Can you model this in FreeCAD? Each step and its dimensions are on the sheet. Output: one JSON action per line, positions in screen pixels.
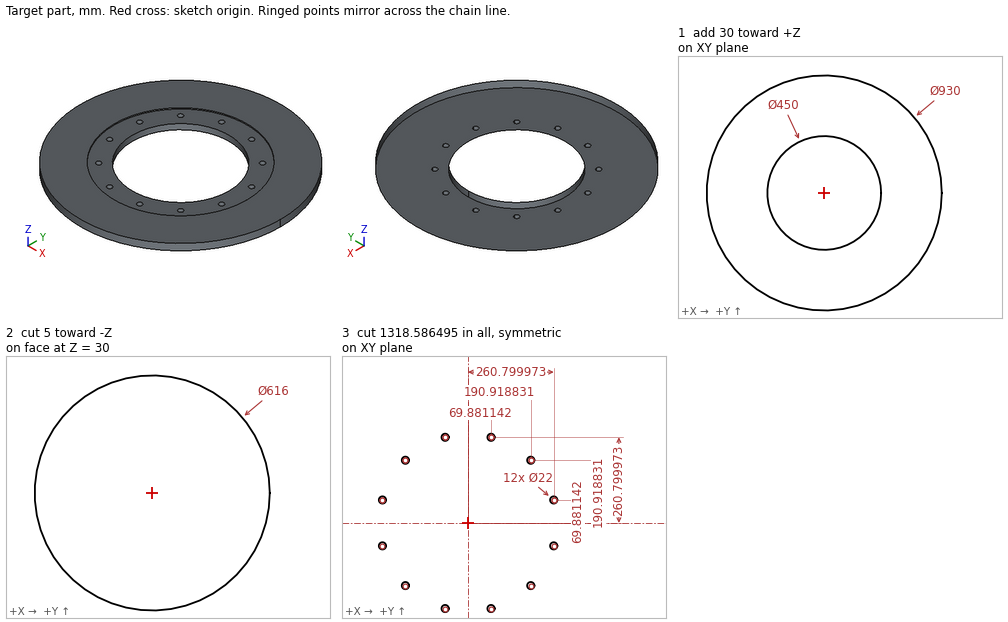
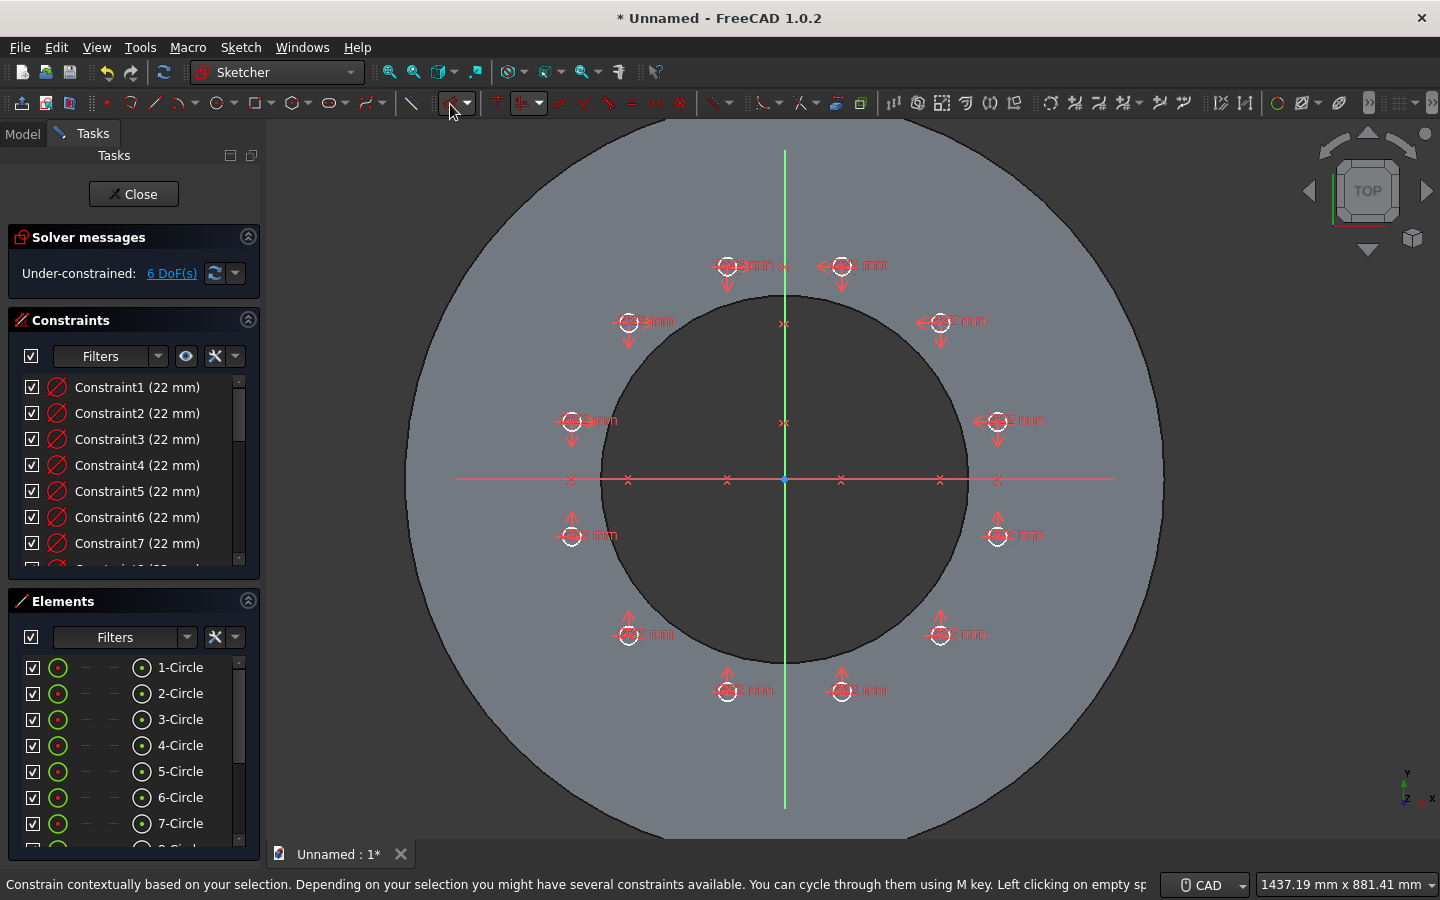
{"action": "left_click", "coordinate": [998, 422]}
{"action": "left_click", "coordinate": [1032, 451]}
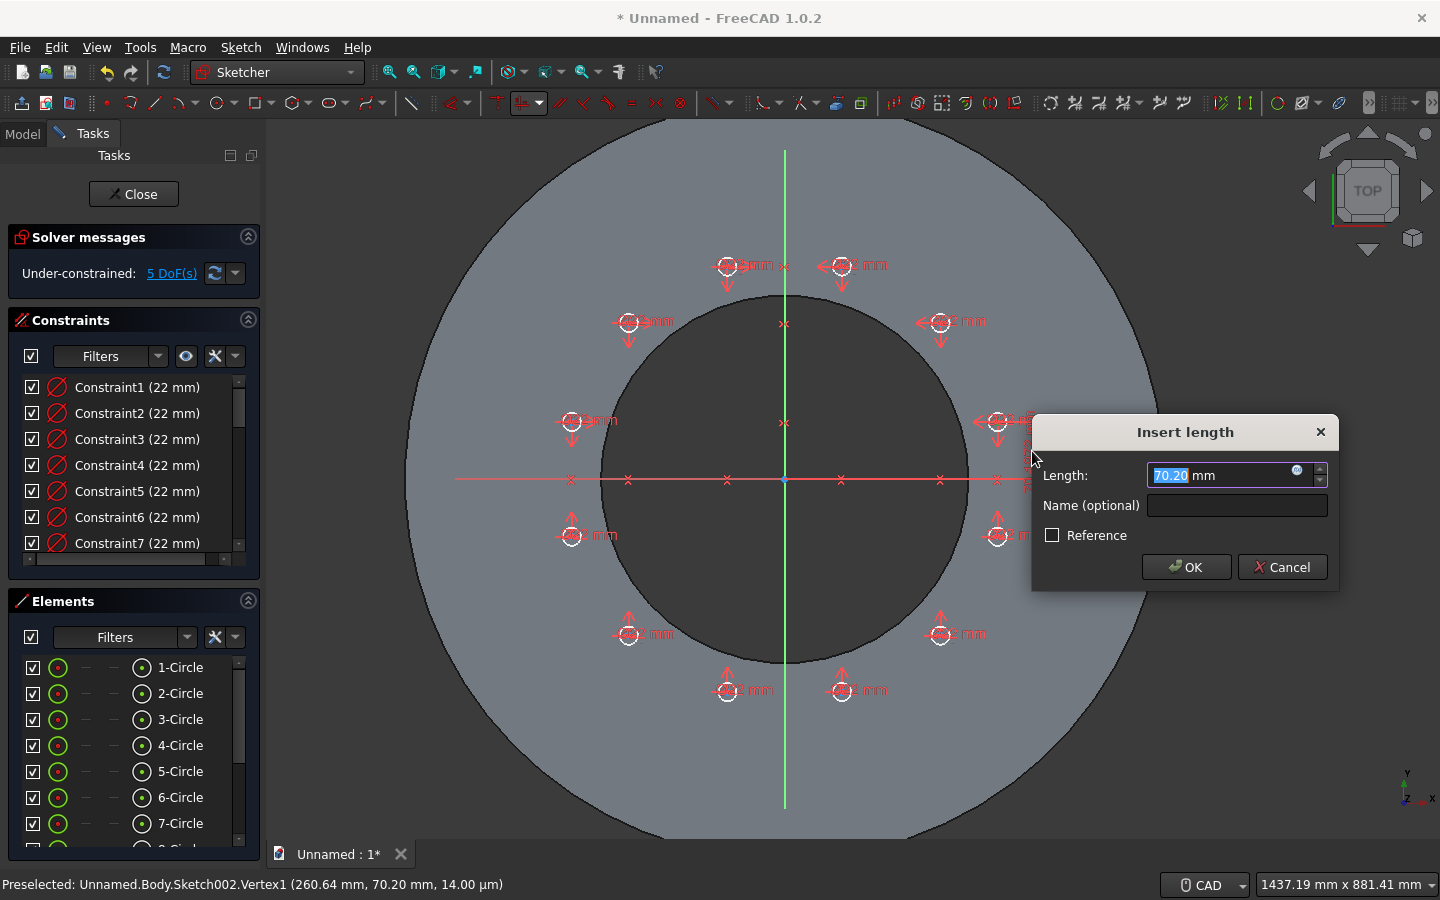
{"action": "type", "text": "69.881142"}
{"action": "key", "text": "Return"}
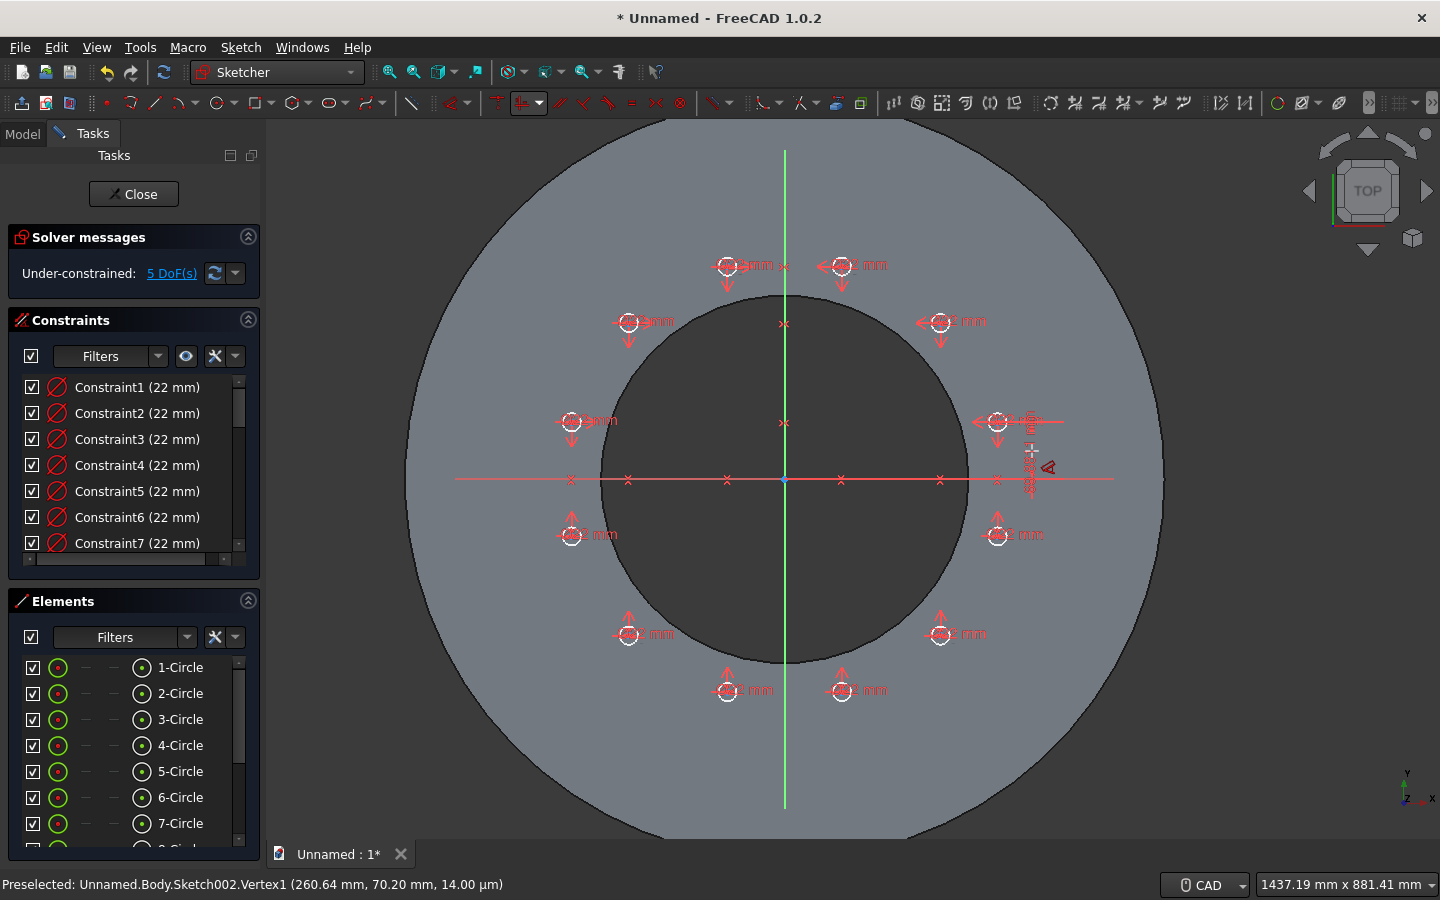
{"action": "left_click", "coordinate": [842, 267]}
{"action": "left_click", "coordinate": [813, 233]}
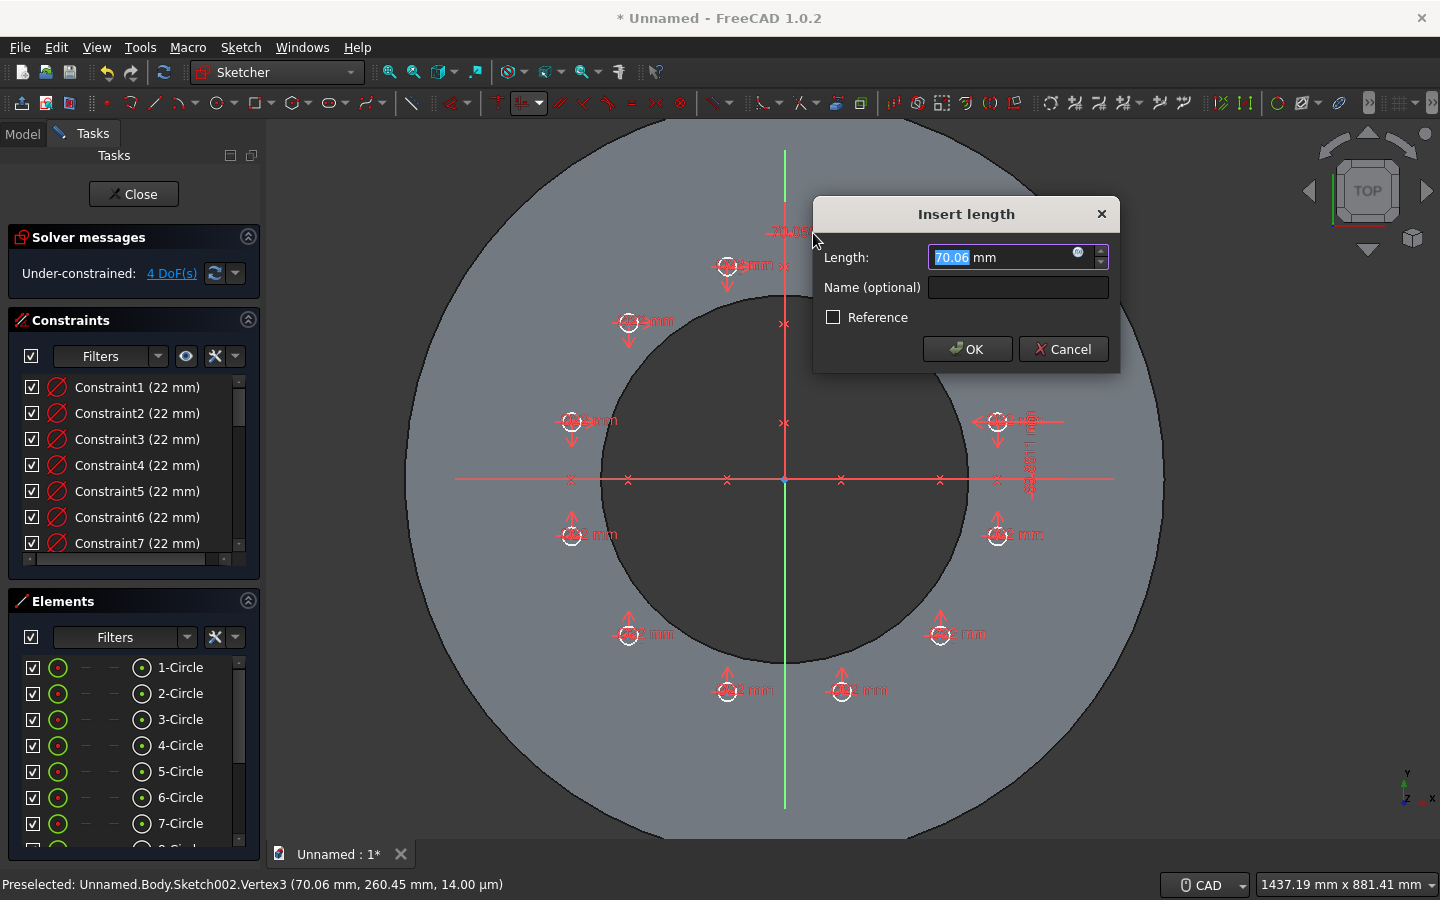
{"action": "type", "text": "69.881142"}
{"action": "key", "text": "Return"}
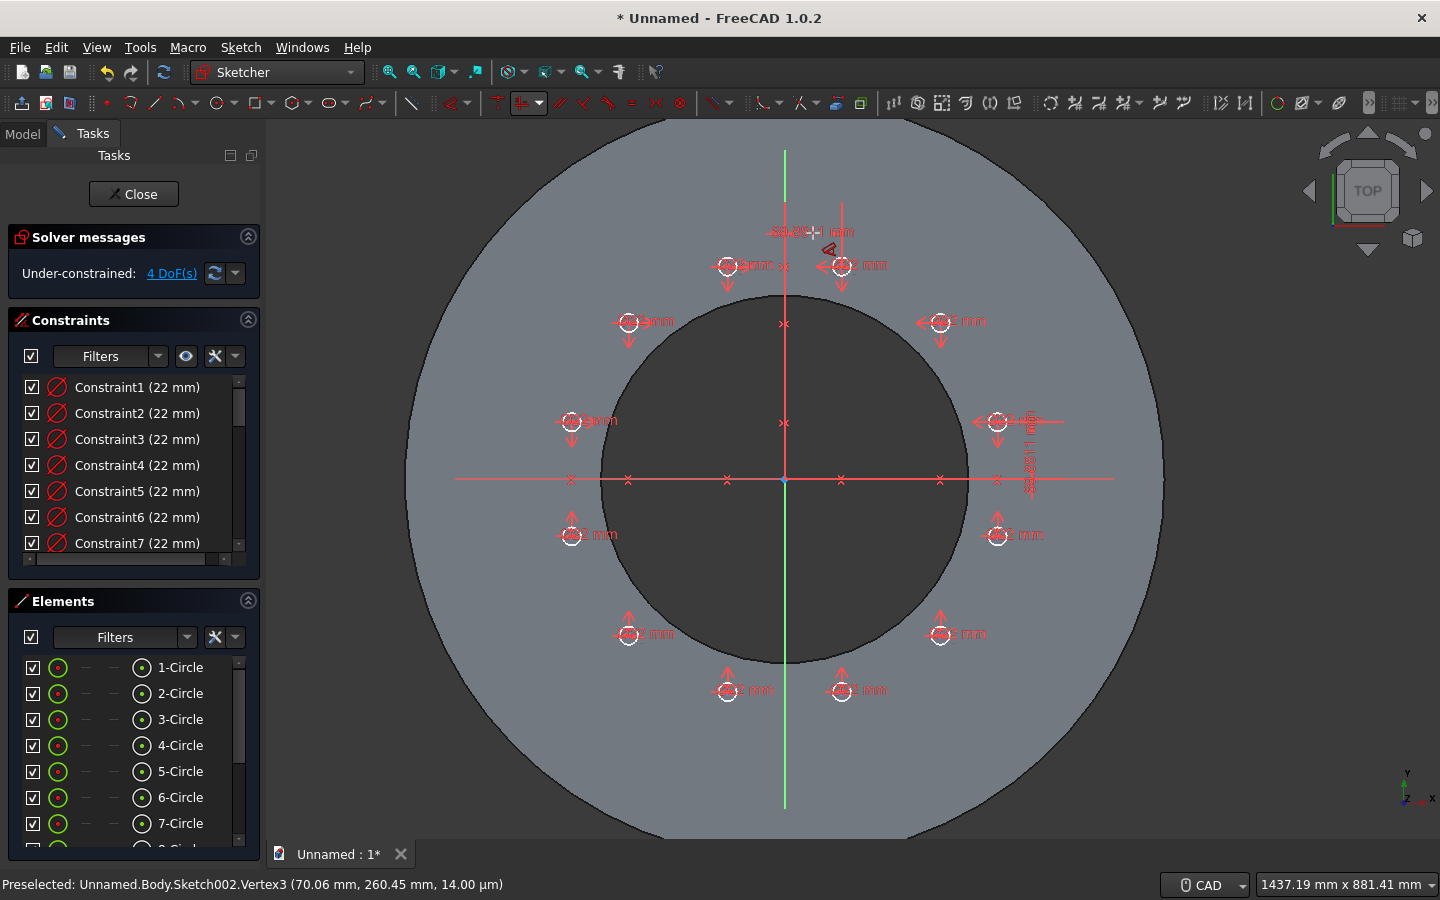
{"action": "left_click", "coordinate": [998, 422]}
{"action": "left_click", "coordinate": [891, 388]}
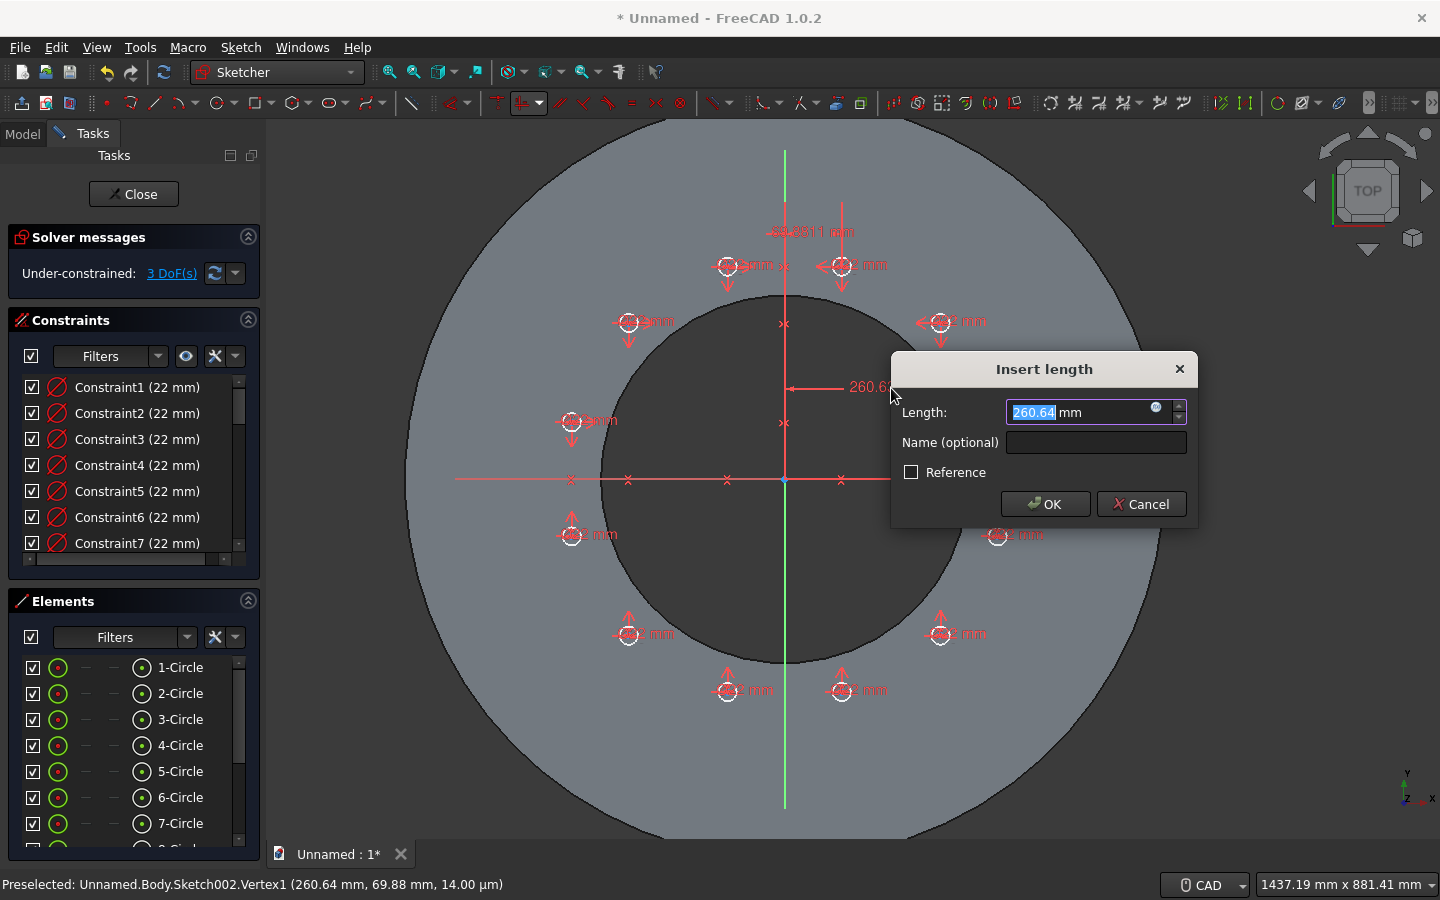
{"action": "type", "text": "260.799973"}
{"action": "key", "text": "Return"}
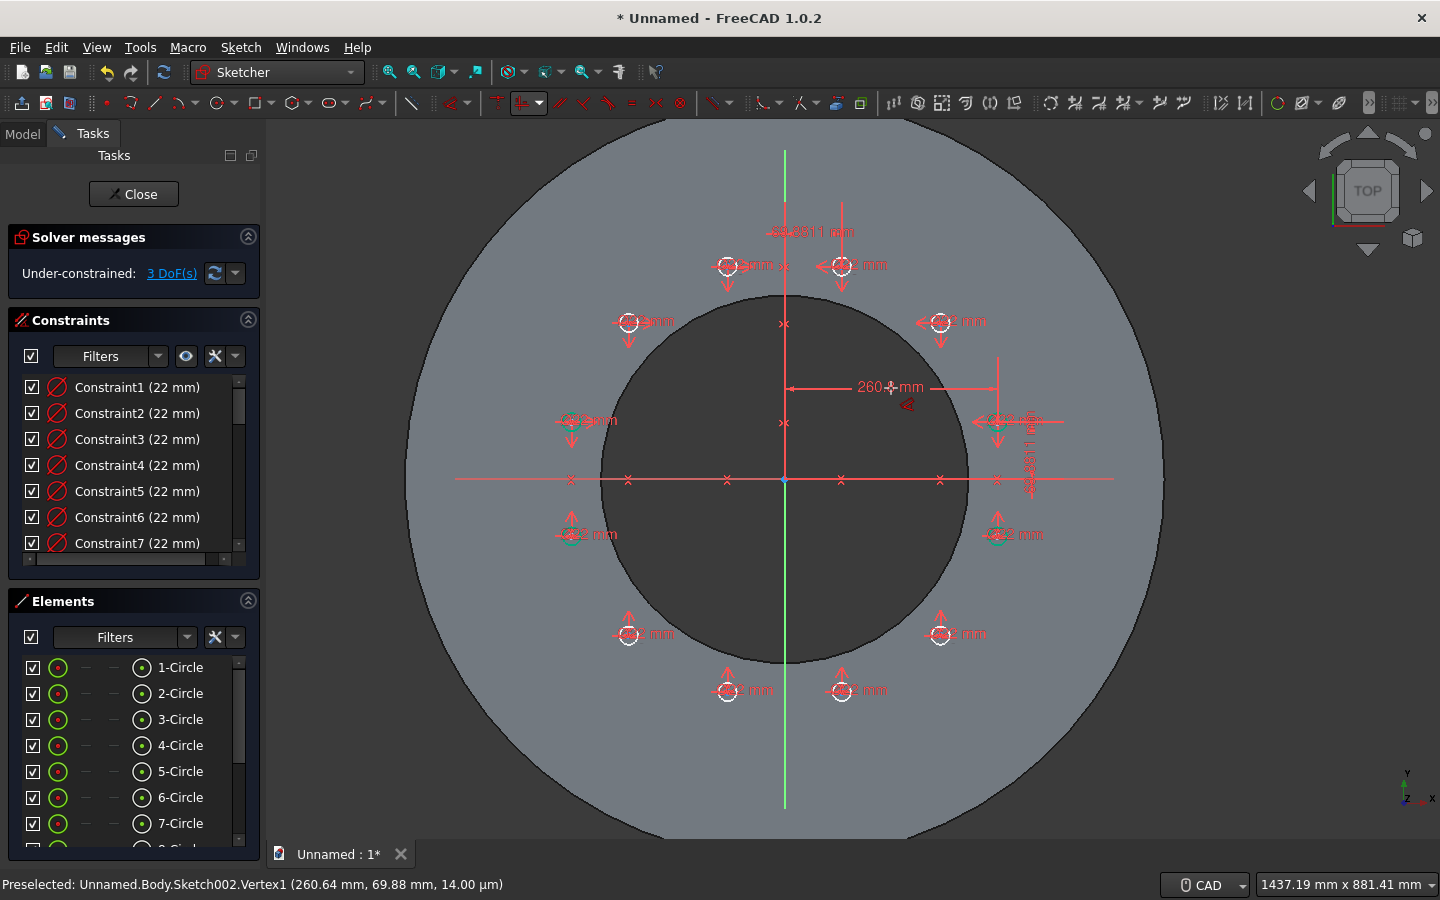
{"action": "left_click", "coordinate": [941, 323]}
{"action": "left_click", "coordinate": [863, 289]}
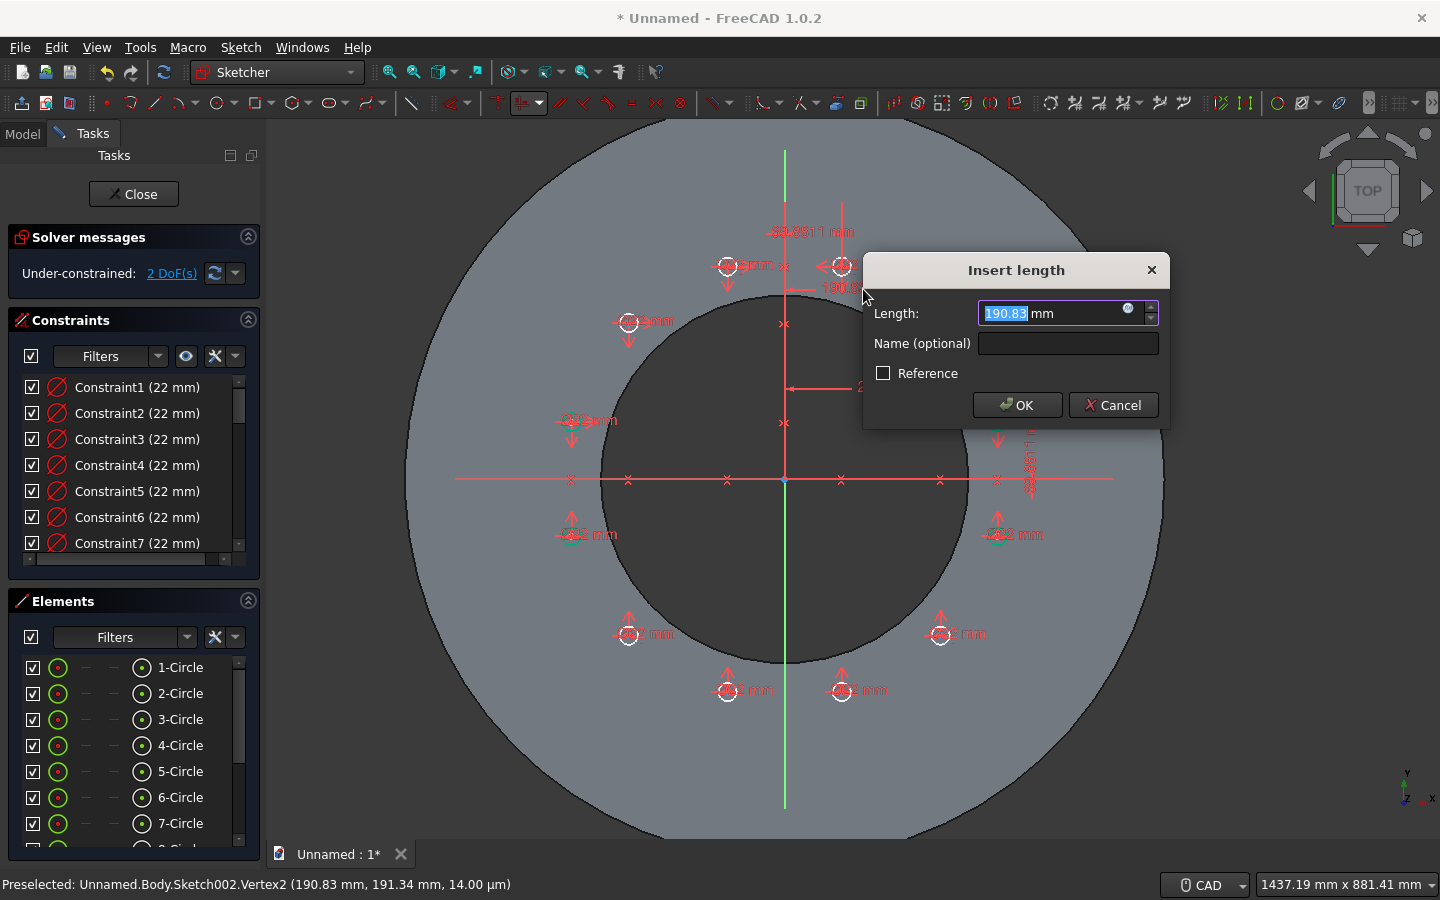
{"action": "type", "text": "190.918831"}
{"action": "key", "text": "Return"}